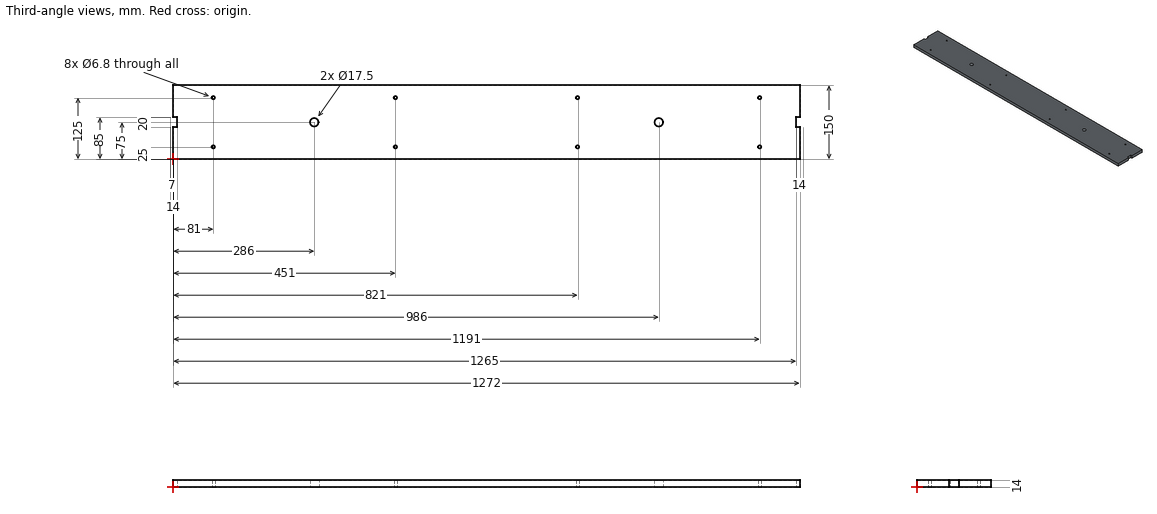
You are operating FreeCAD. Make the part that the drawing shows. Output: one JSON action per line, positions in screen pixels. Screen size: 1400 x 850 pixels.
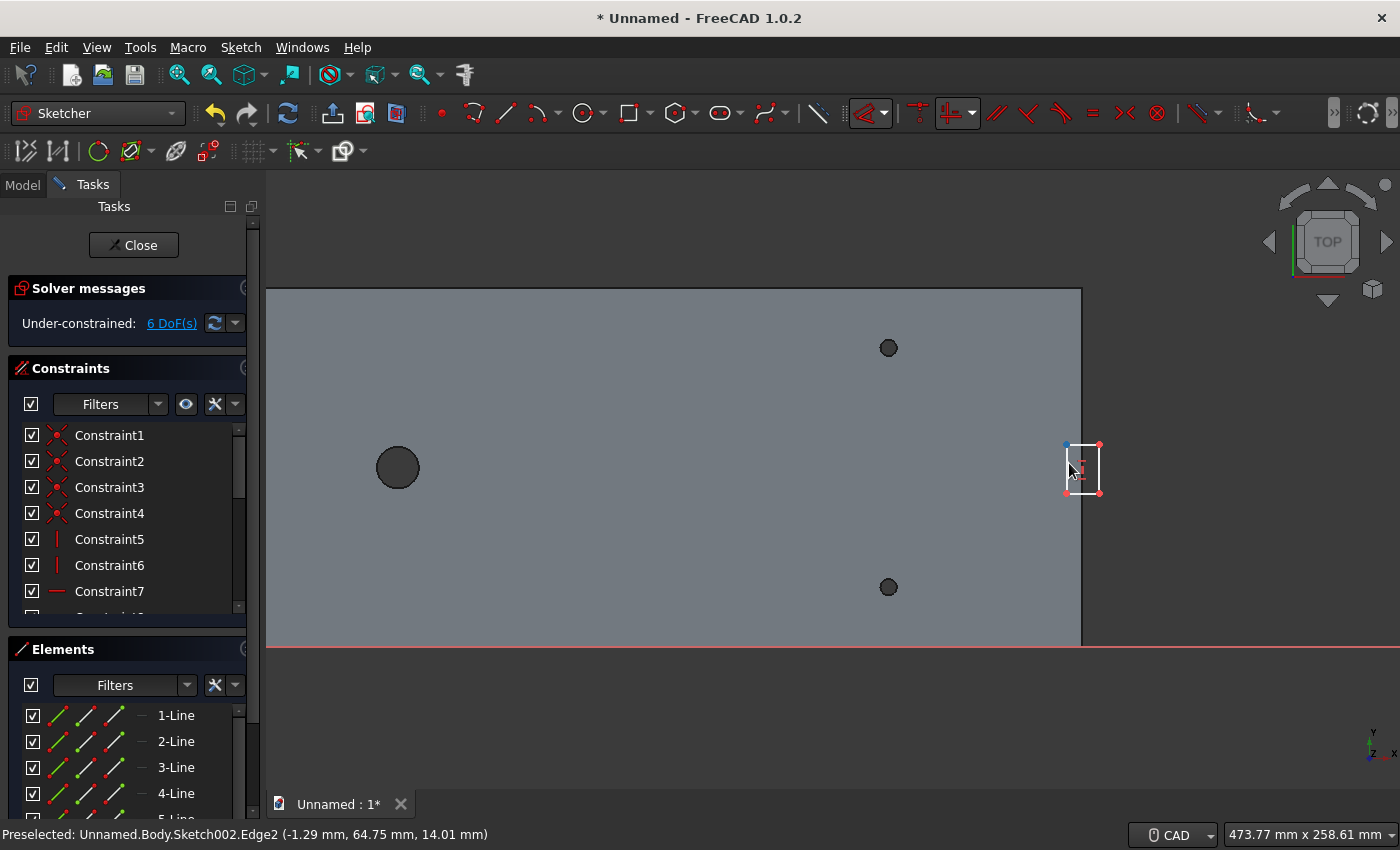
{"action": "left_click", "coordinate": [1067, 459]}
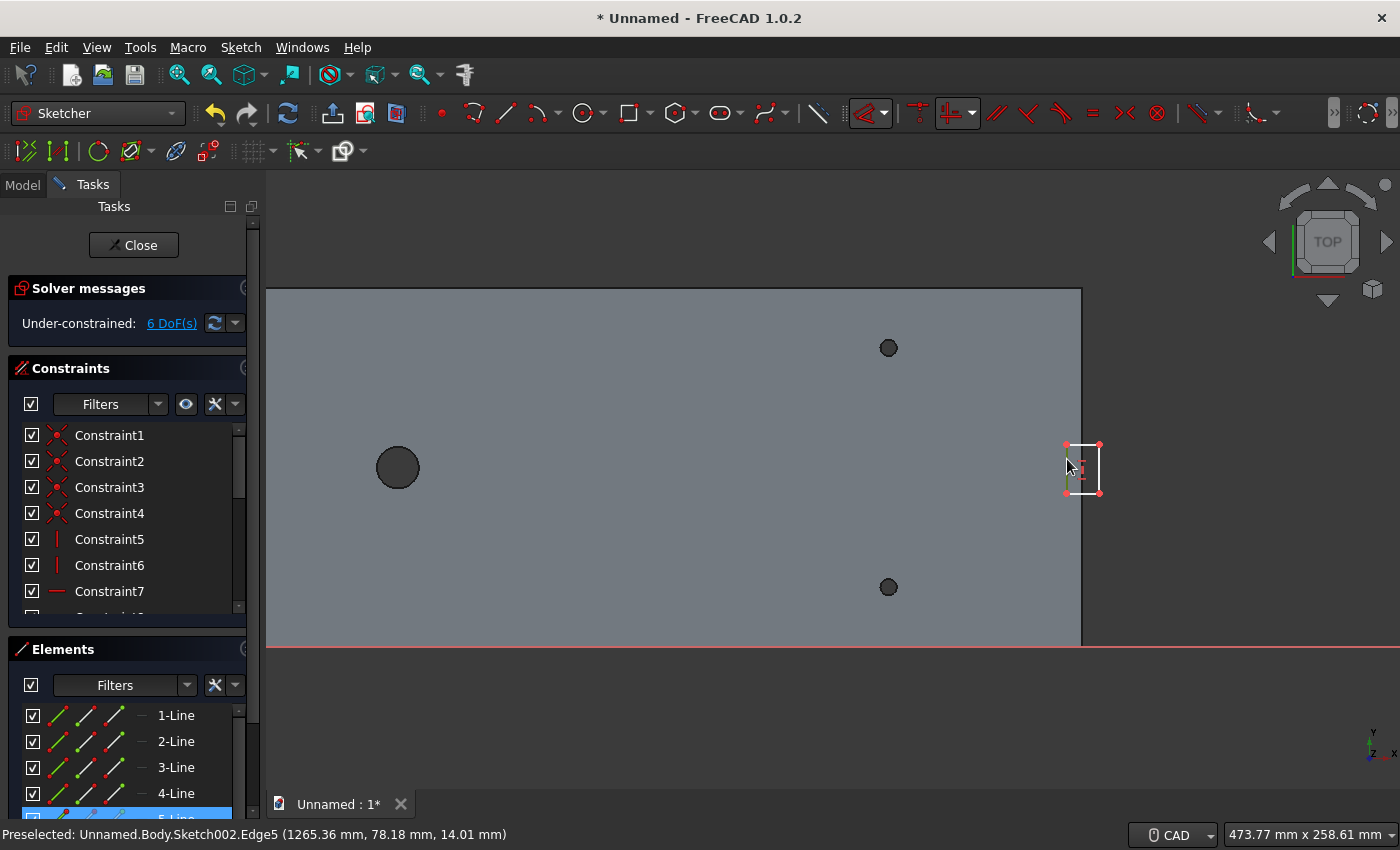
{"action": "left_click", "coordinate": [886, 114]}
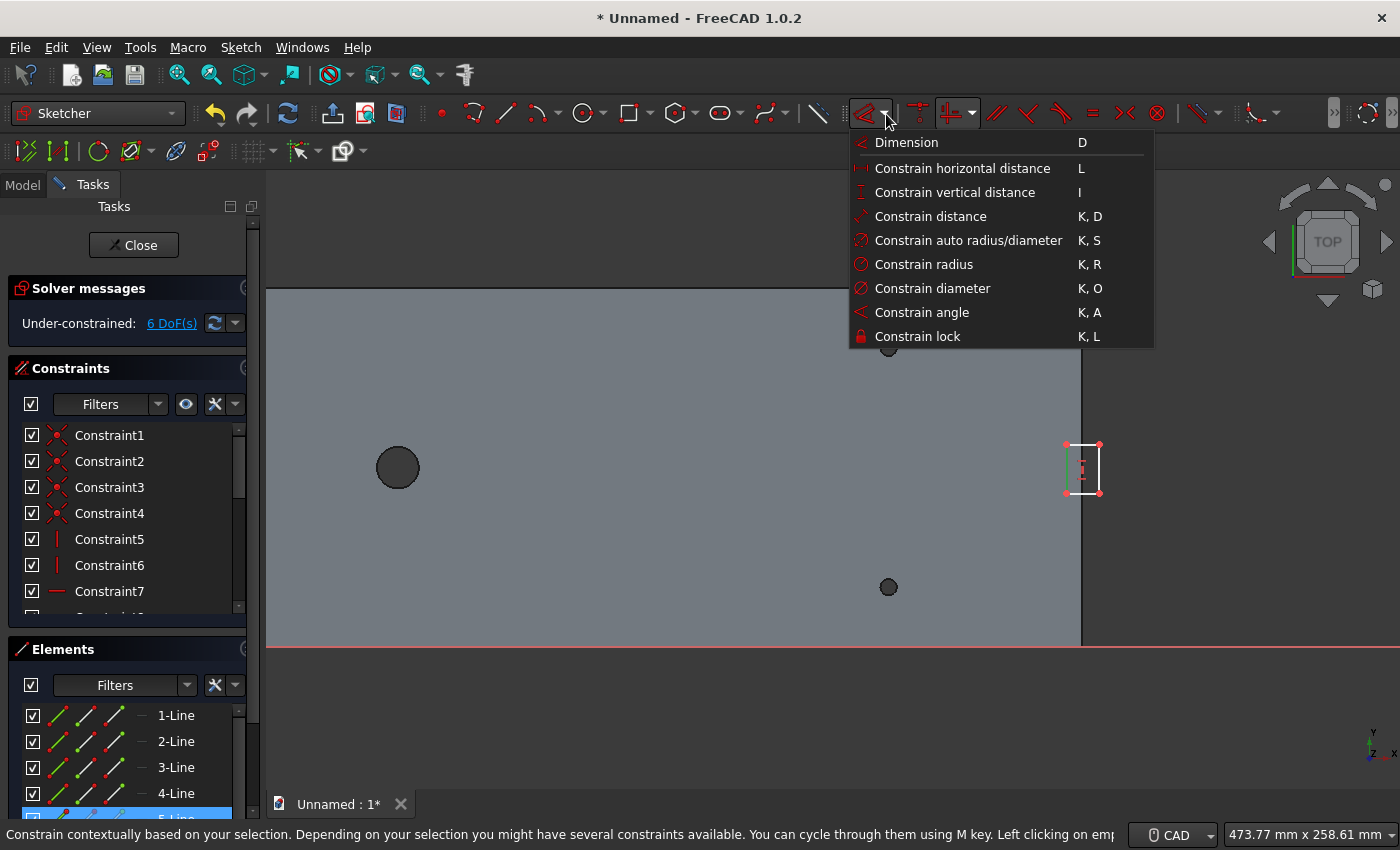
{"action": "left_click", "coordinate": [1002, 192]}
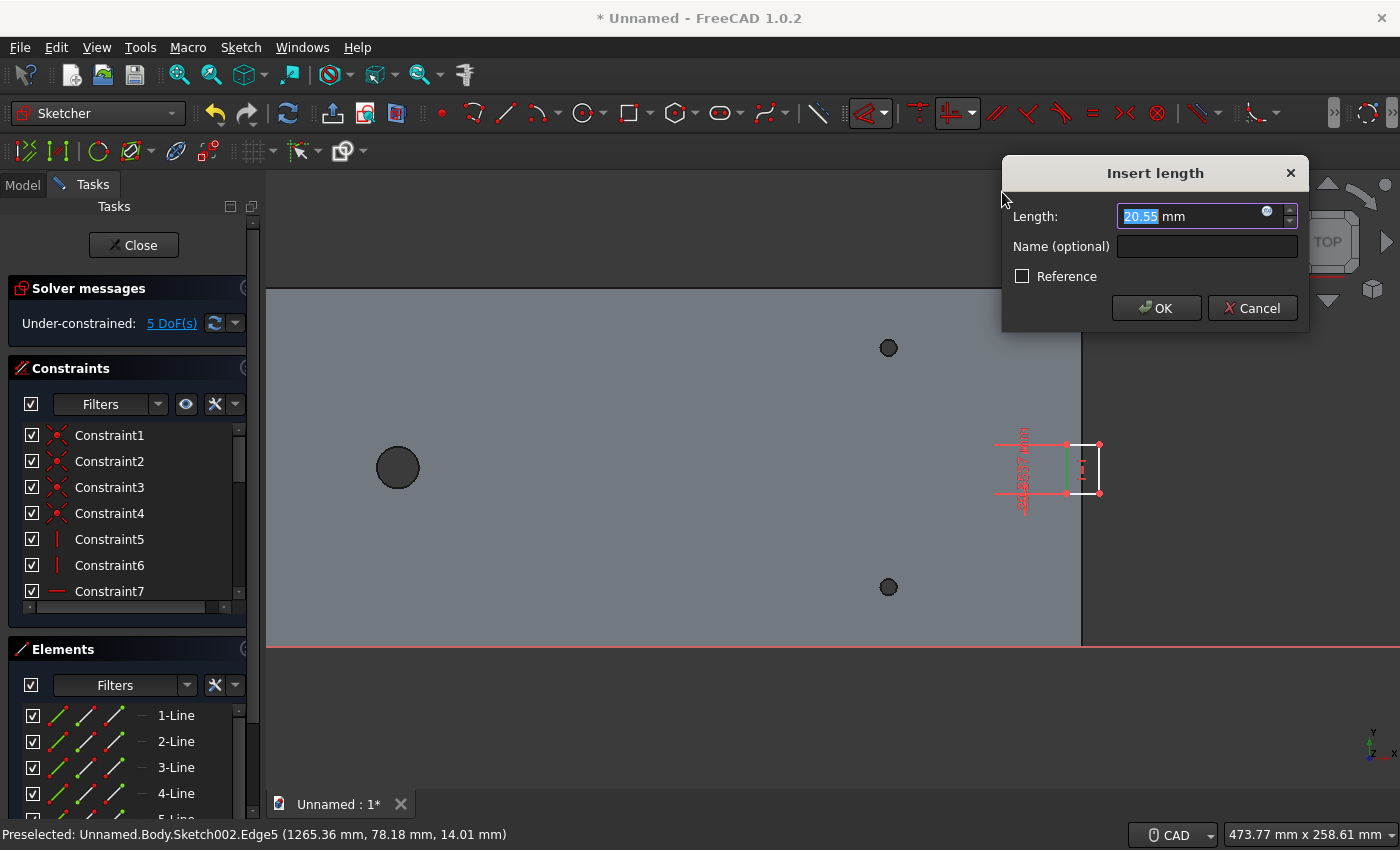
{"action": "type", "text": "20"}
{"action": "key", "text": "Return"}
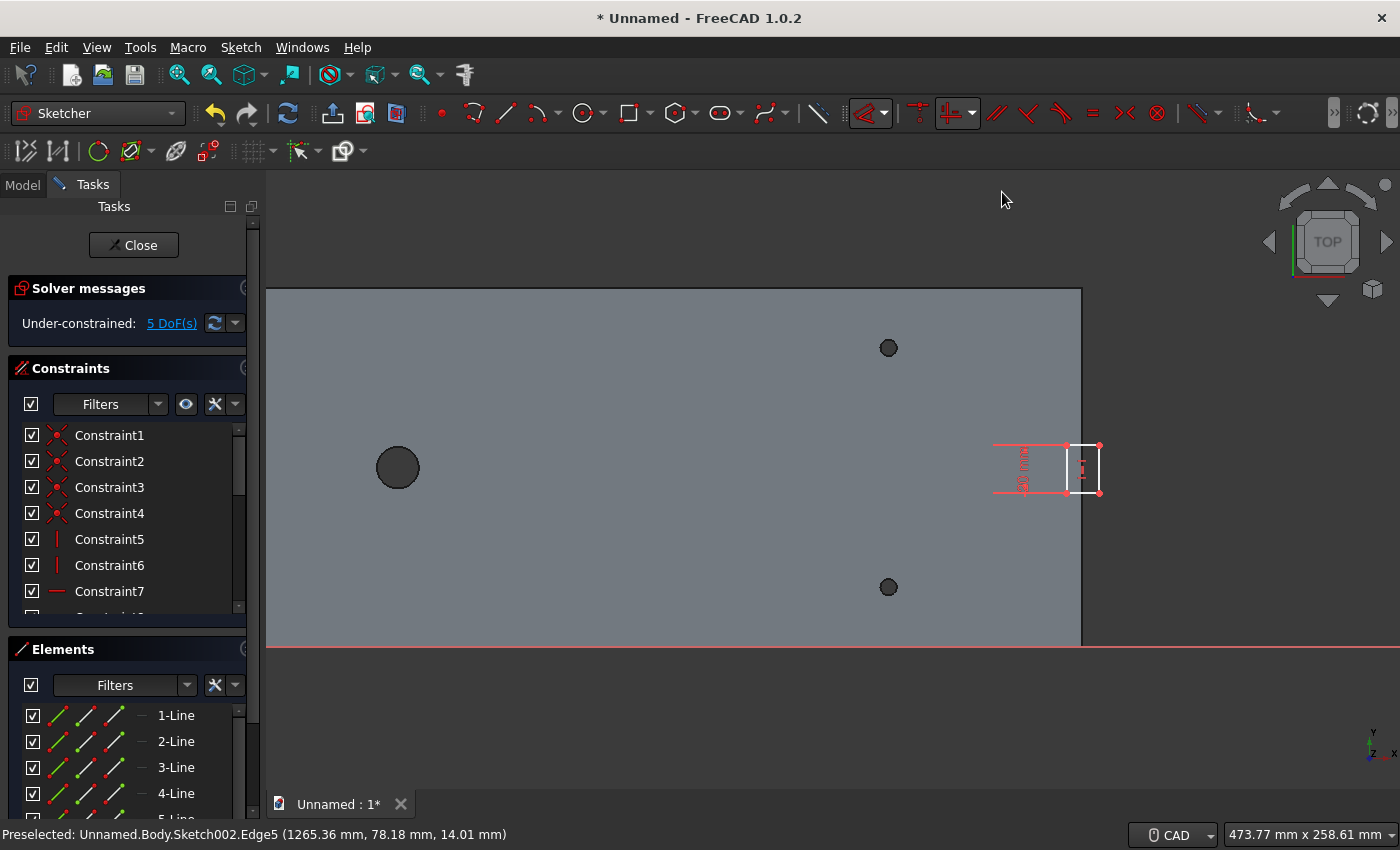
{"action": "scroll", "coordinate": [1076, 493], "scroll_direction": "up", "scroll_amount": 2}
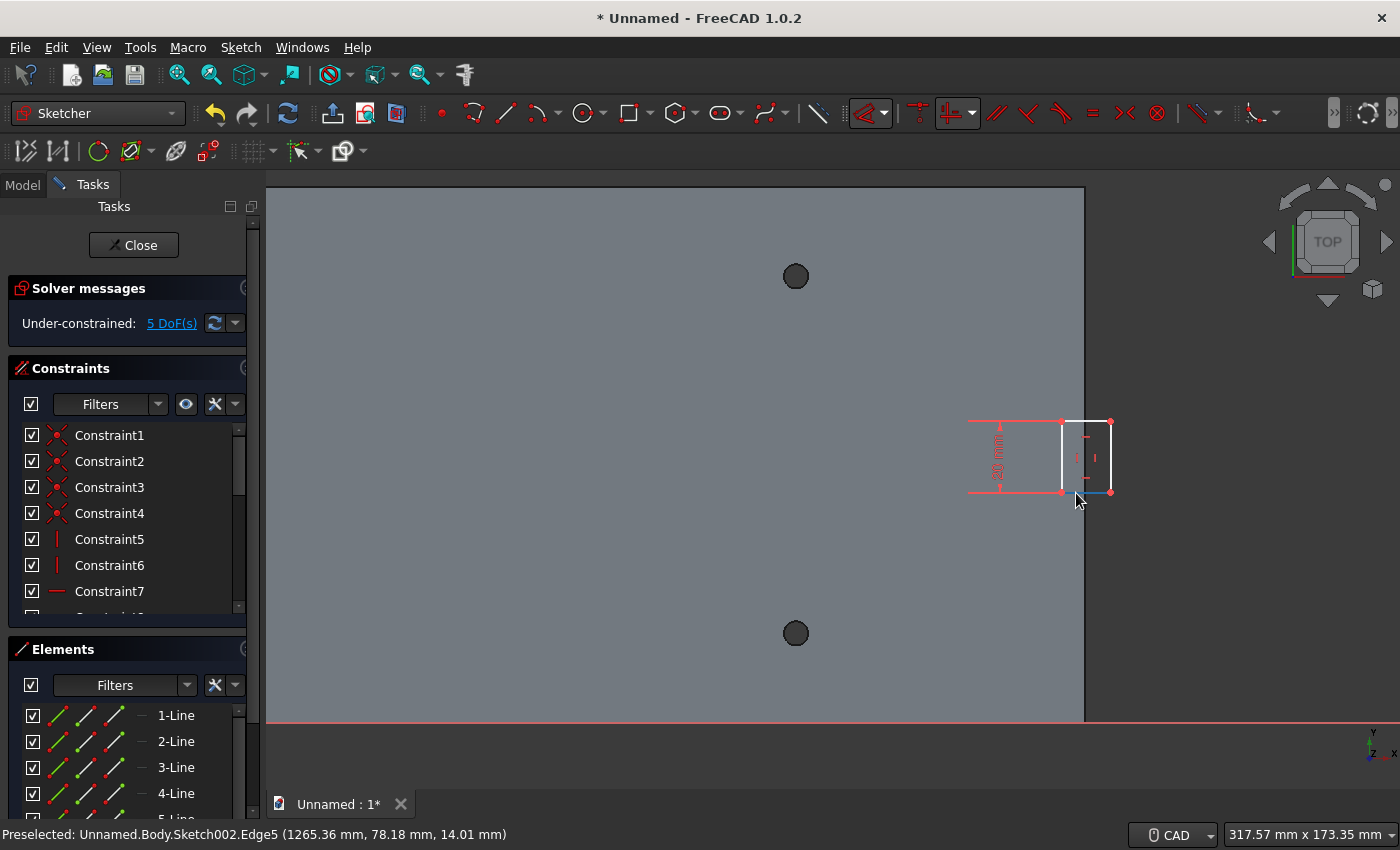
{"action": "left_click", "coordinate": [1076, 493]}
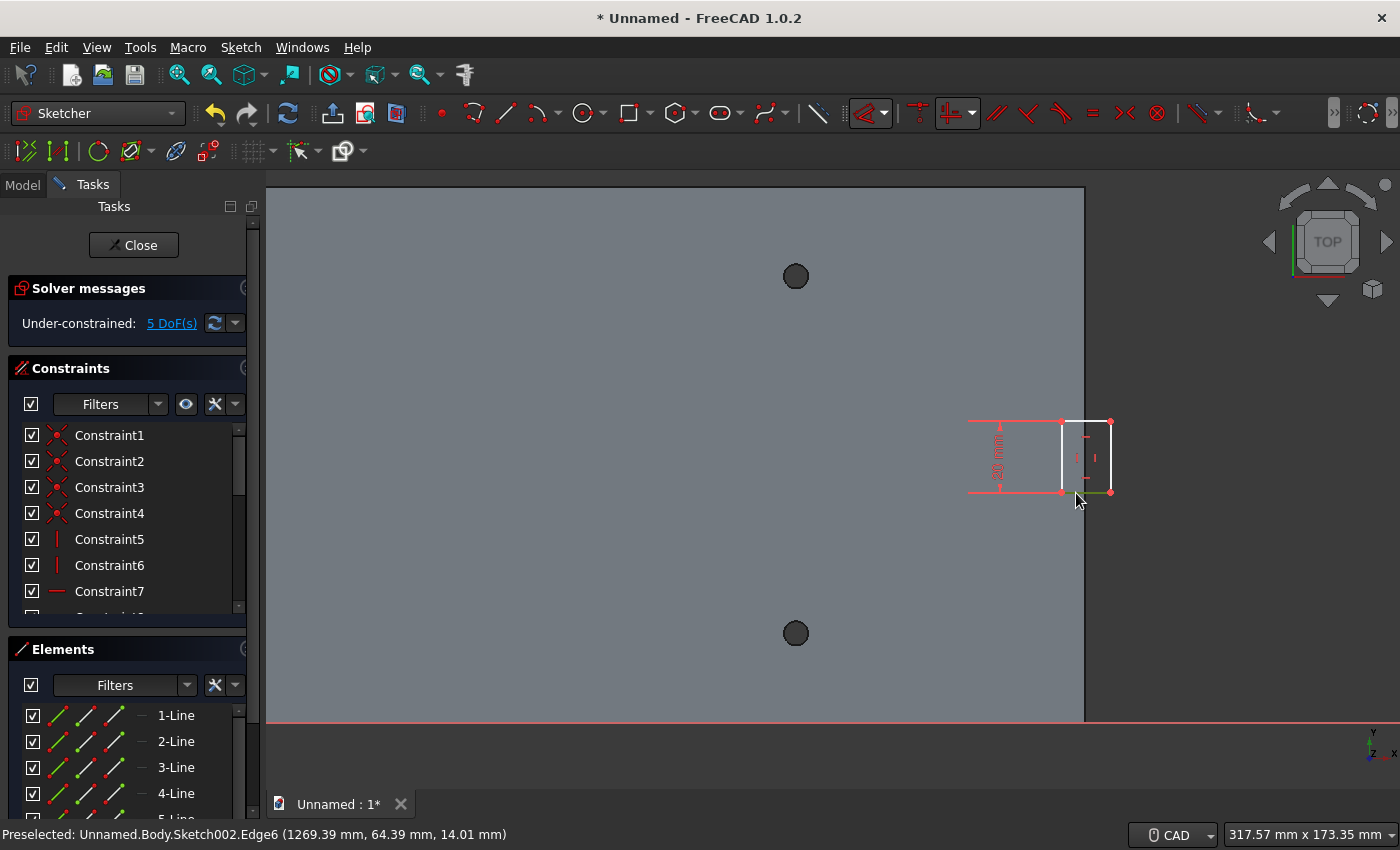
{"action": "left_click", "coordinate": [886, 114]}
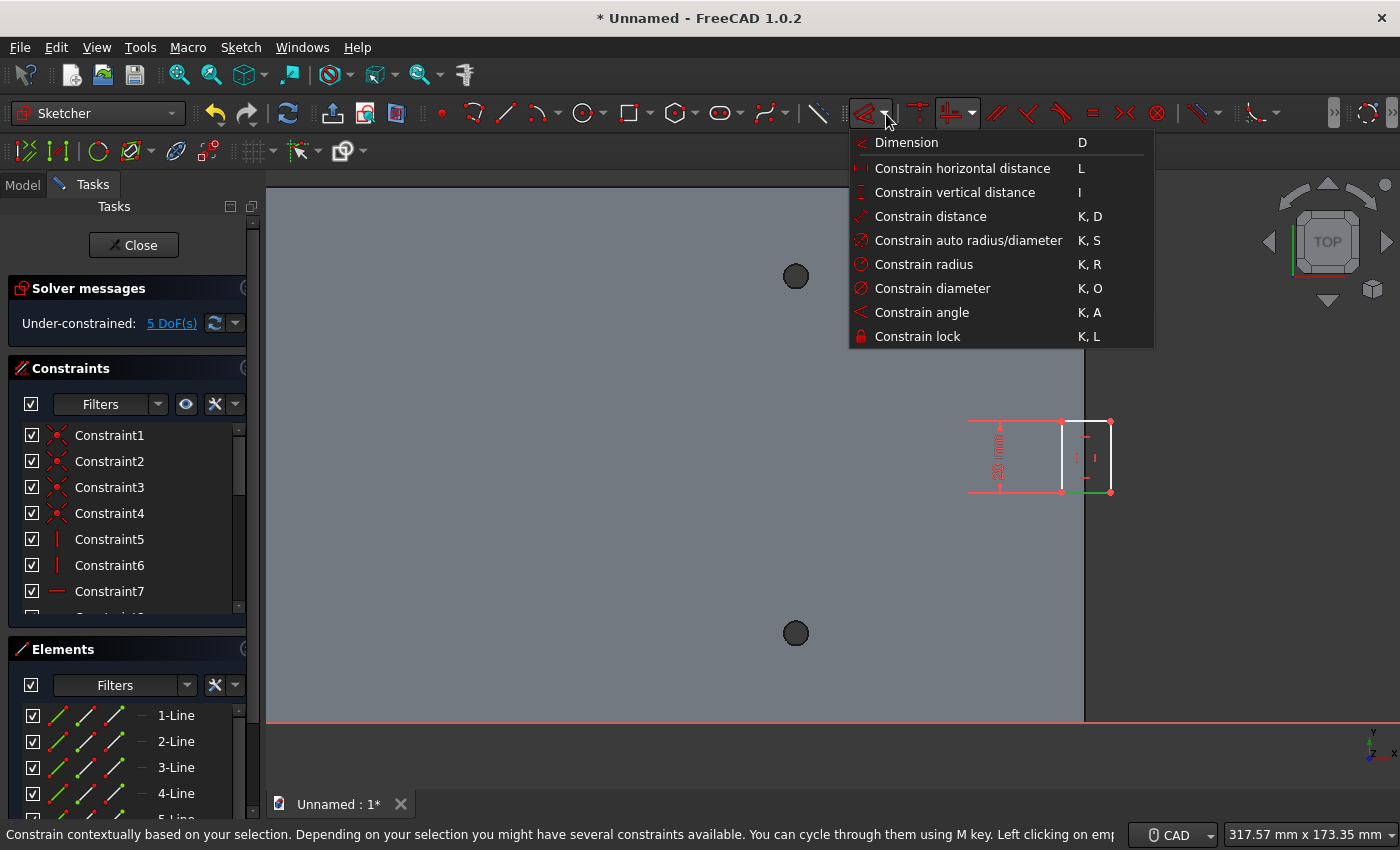
{"action": "left_click", "coordinate": [1002, 168]}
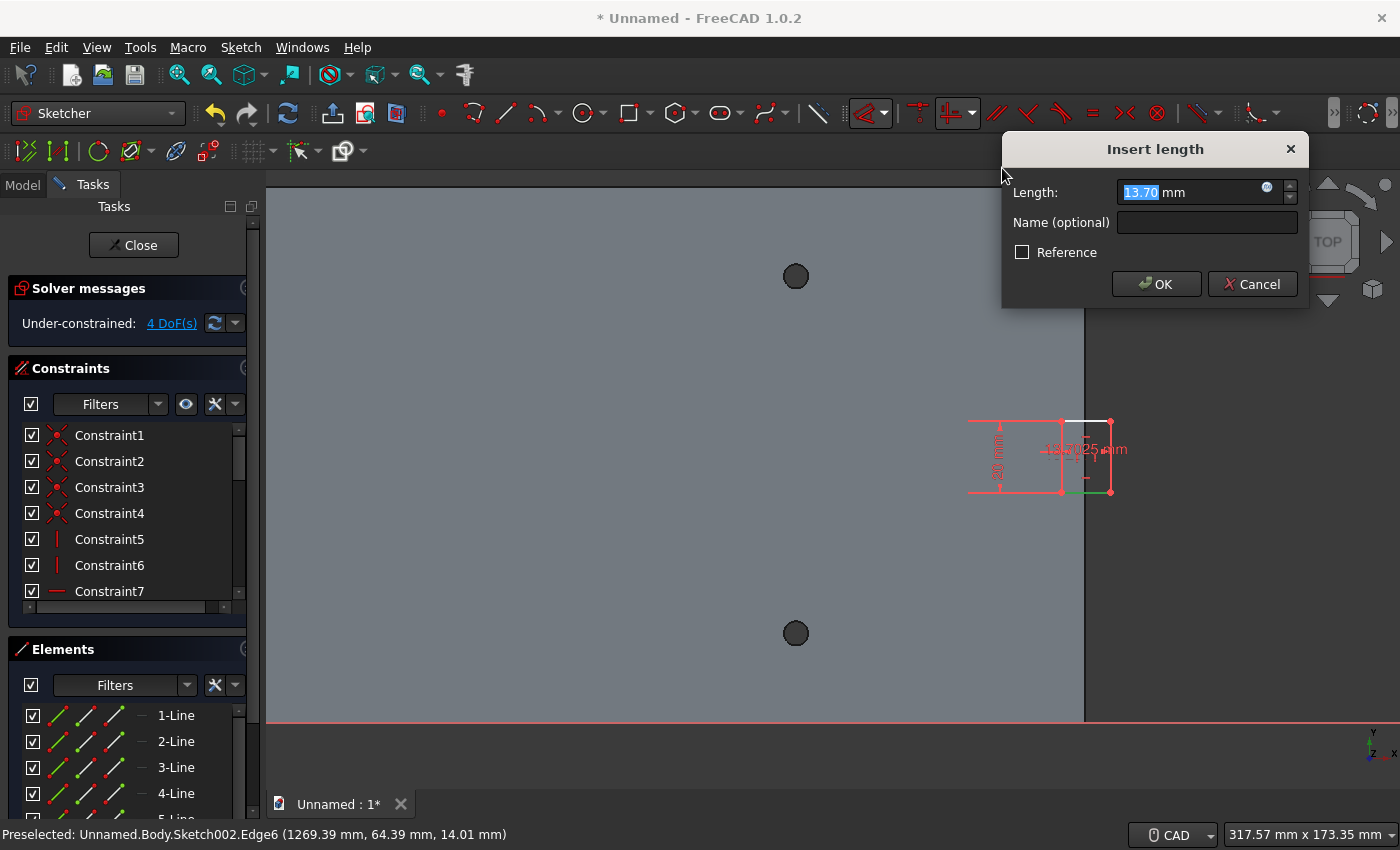
{"action": "type", "text": "14"}
{"action": "key", "text": "Return"}